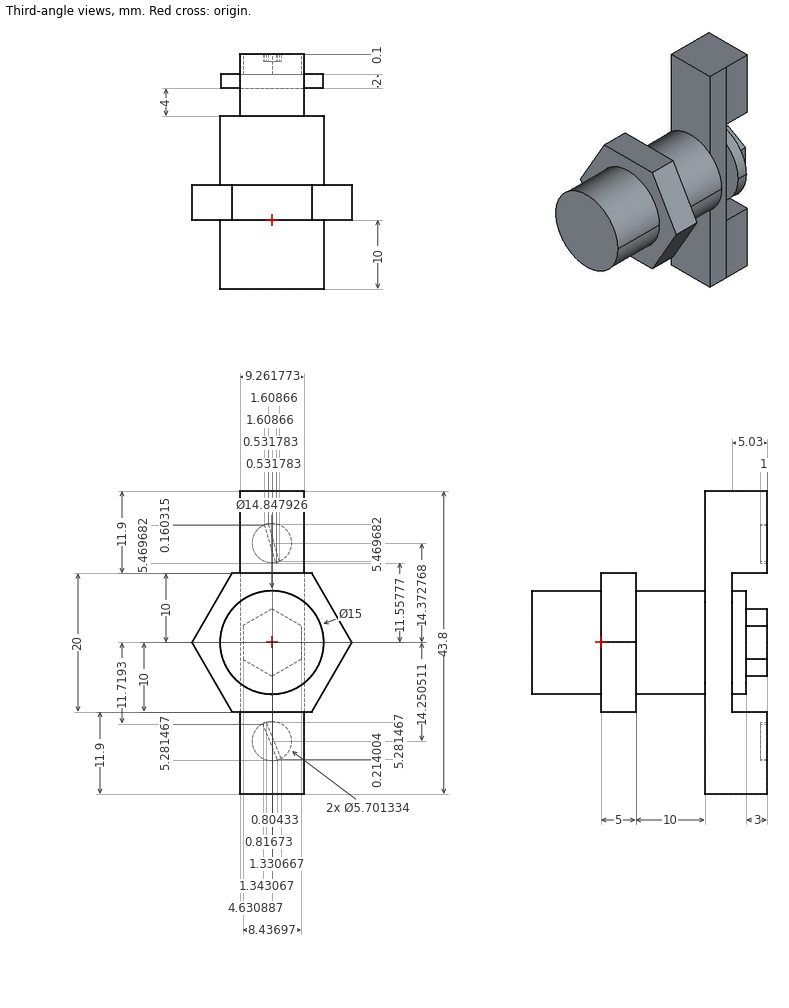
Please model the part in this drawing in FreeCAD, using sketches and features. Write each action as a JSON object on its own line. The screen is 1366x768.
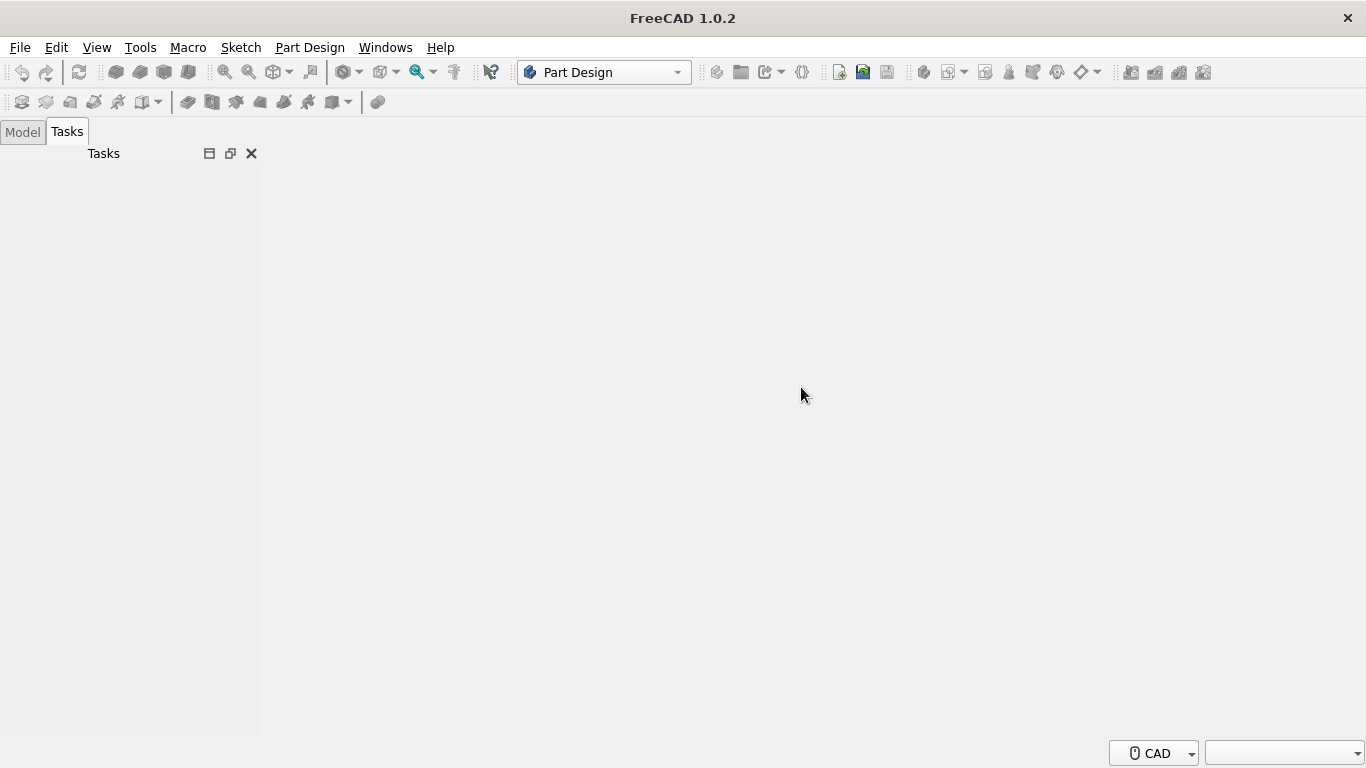
{"action": "left_click", "coordinate": [840, 72]}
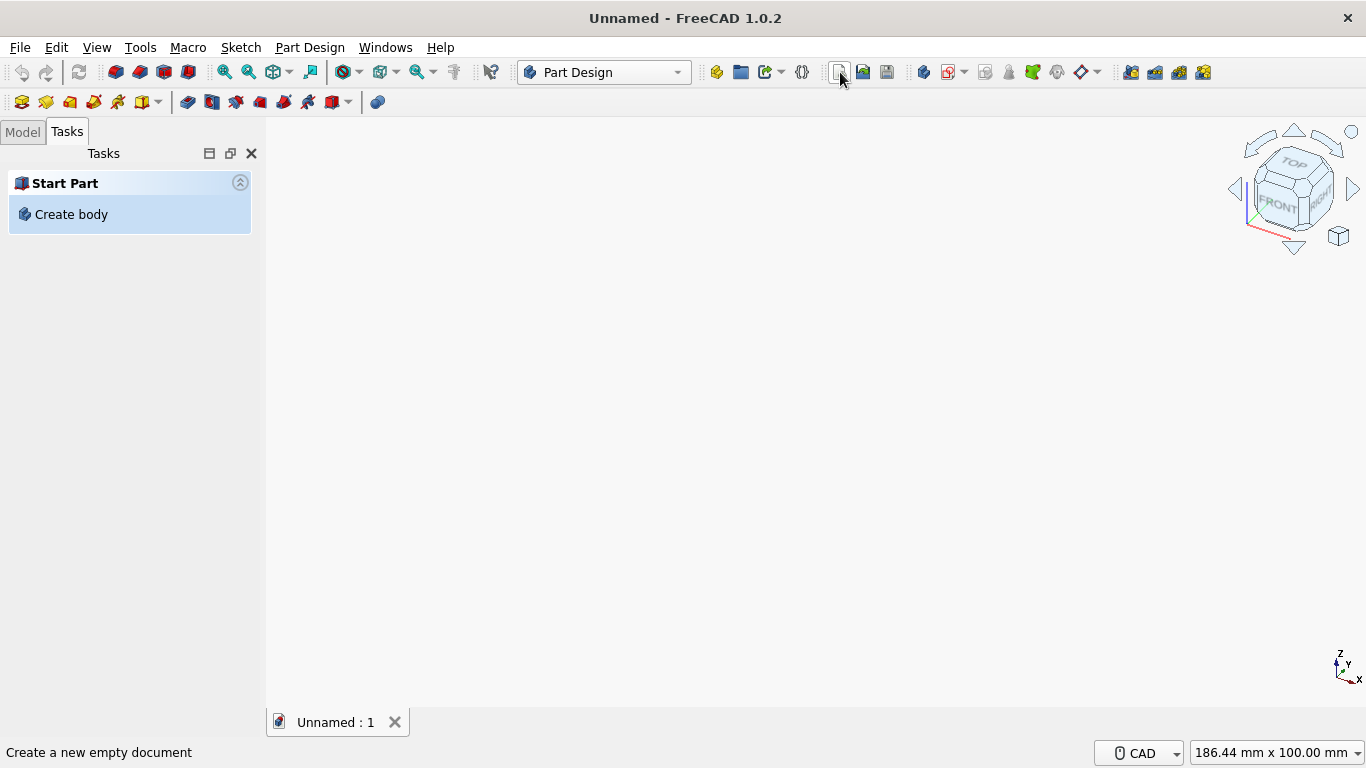
{"action": "left_click", "coordinate": [948, 72]}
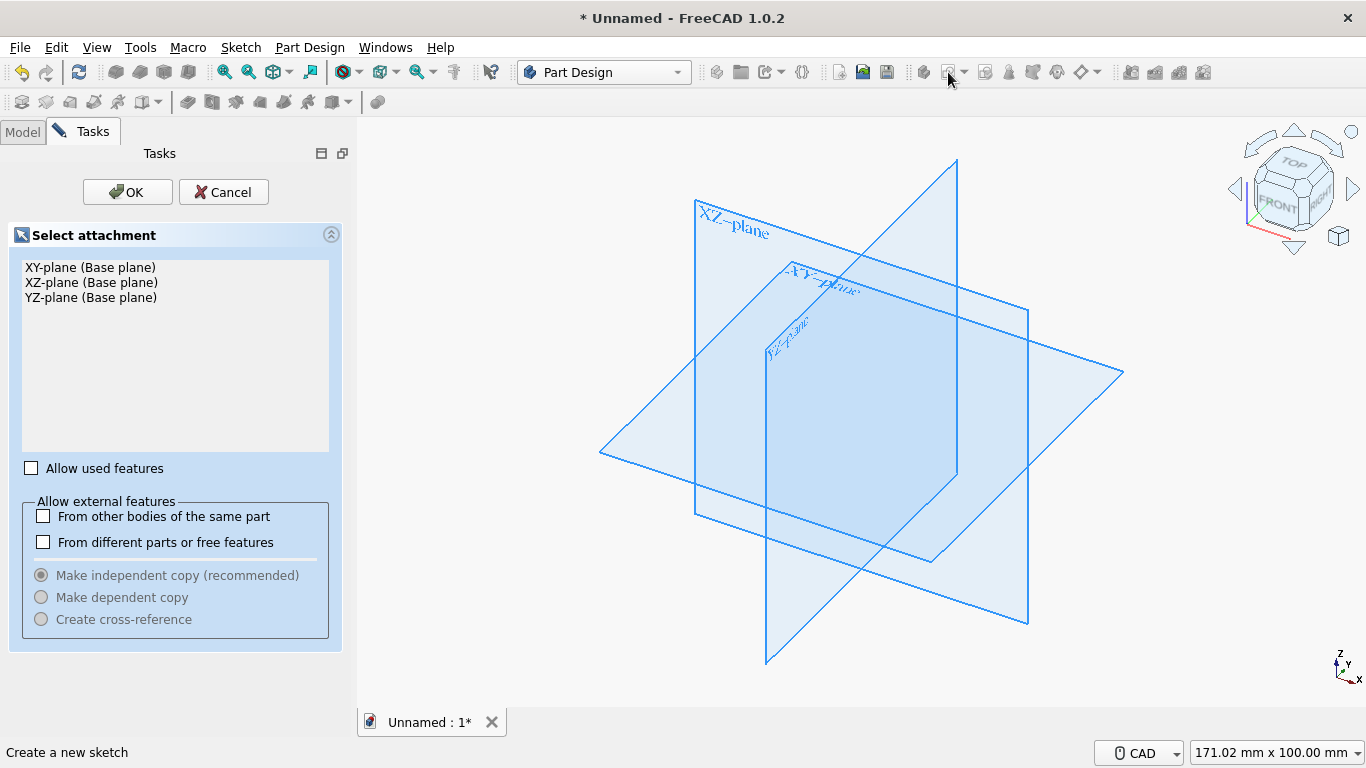
{"action": "left_click", "coordinate": [82, 282]}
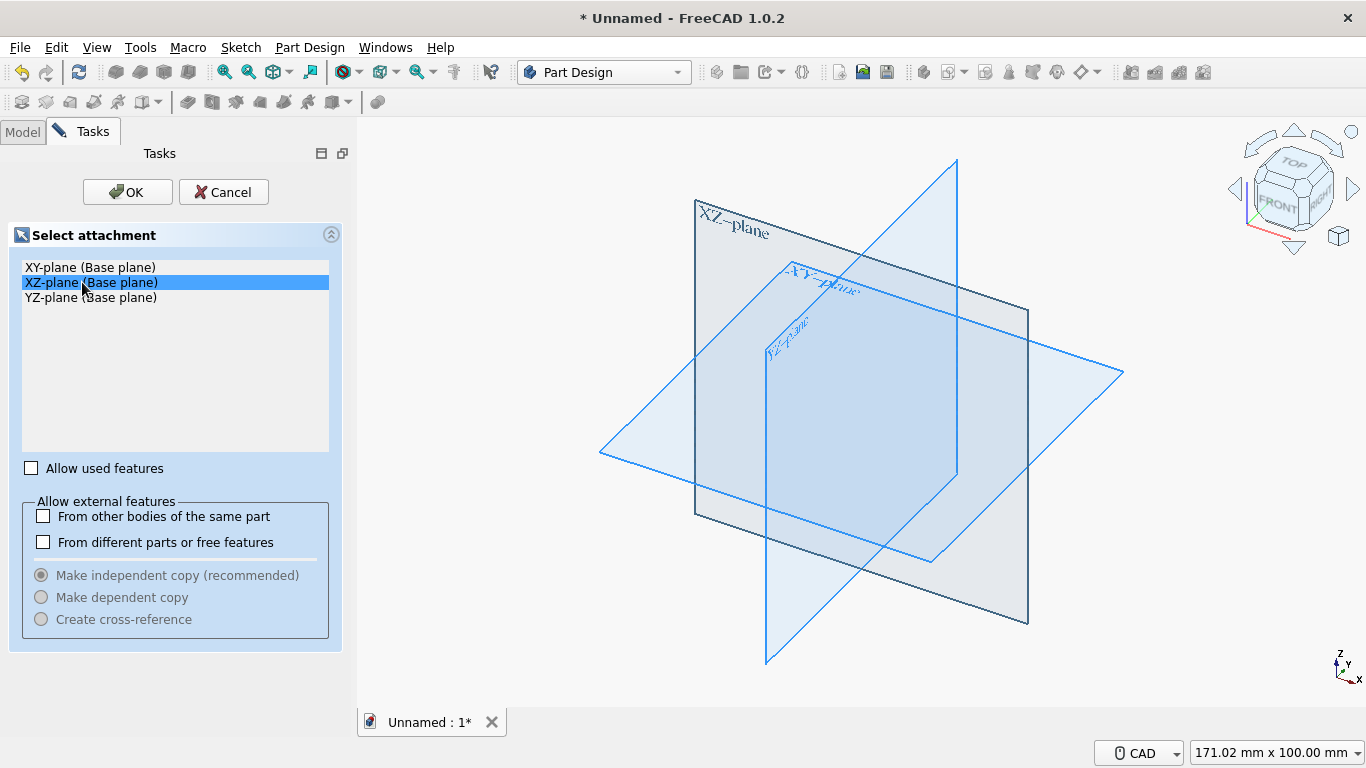
{"action": "left_click", "coordinate": [128, 192]}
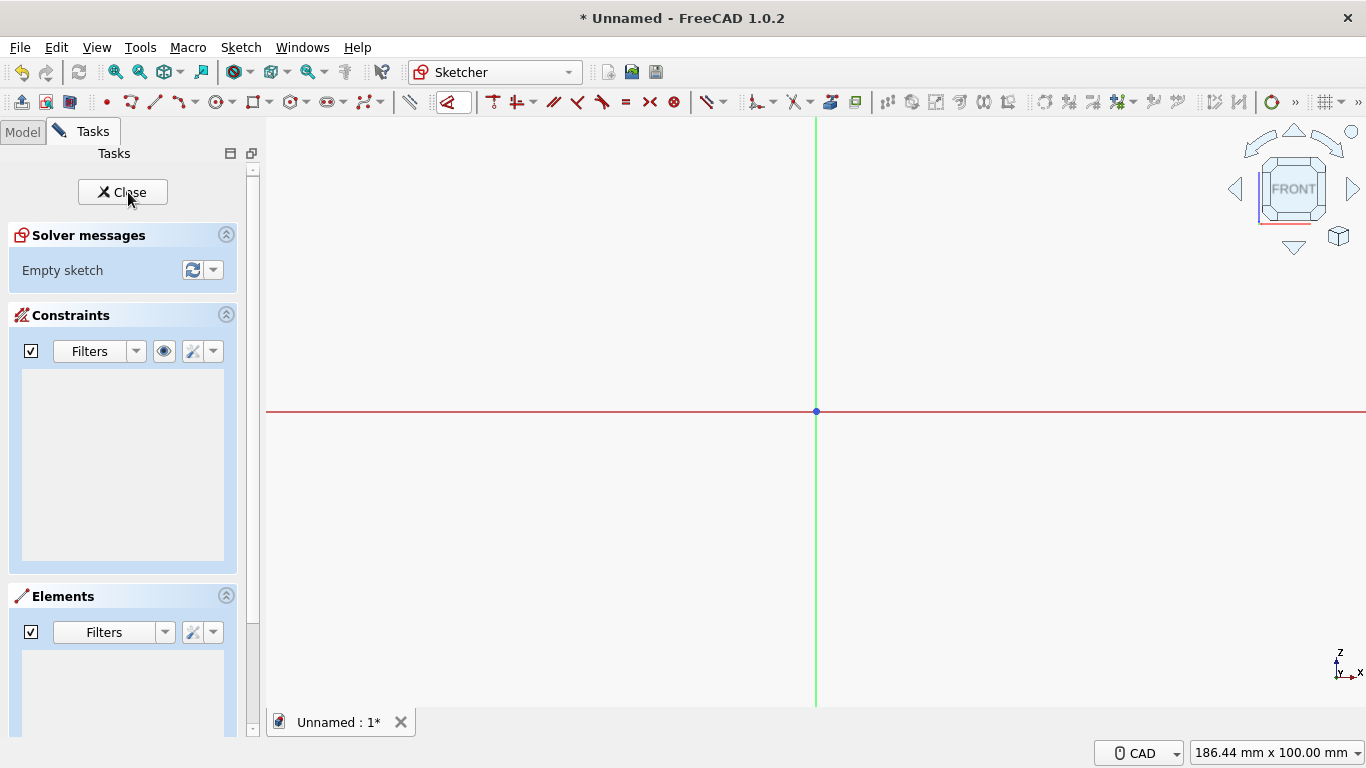
{"action": "scroll", "coordinate": [846, 412], "scroll_direction": "up", "scroll_amount": 6}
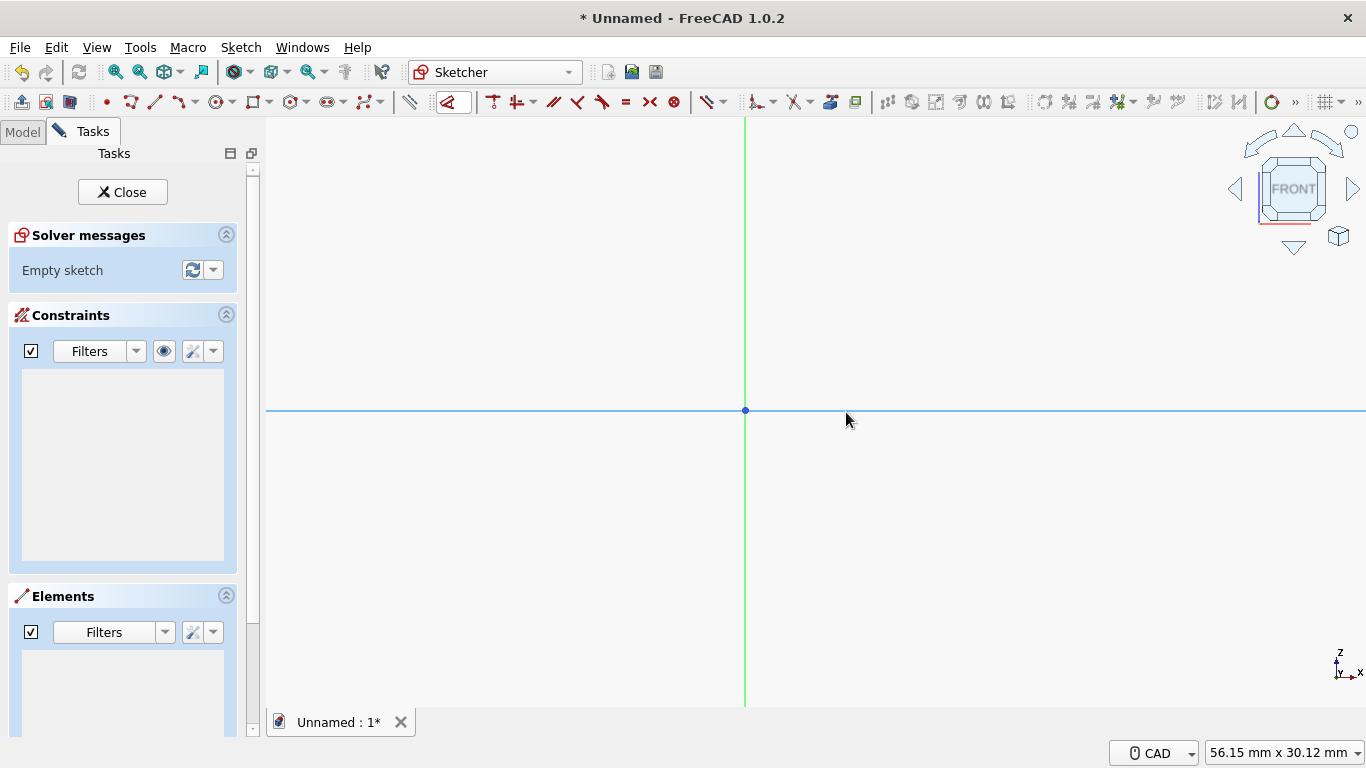
{"action": "left_click", "coordinate": [290, 102]}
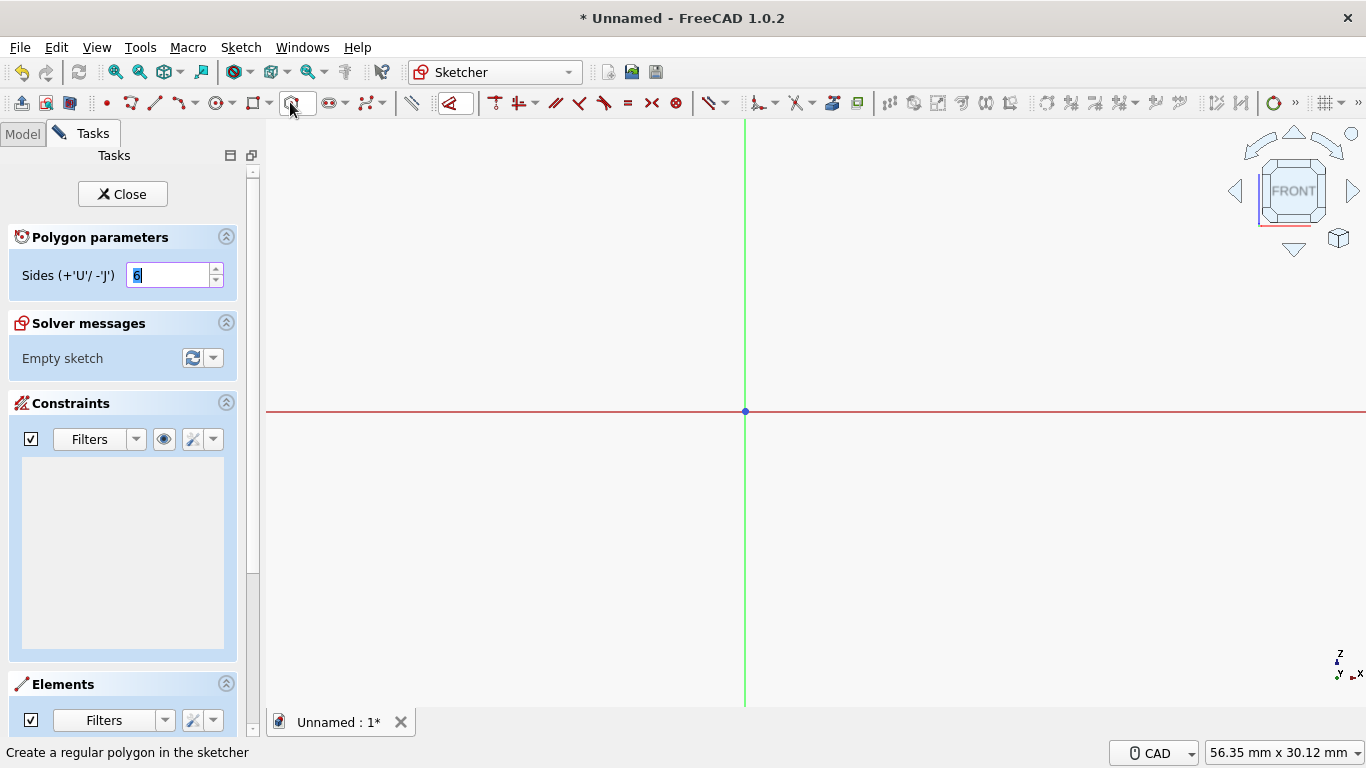
{"action": "left_click", "coordinate": [745, 412]}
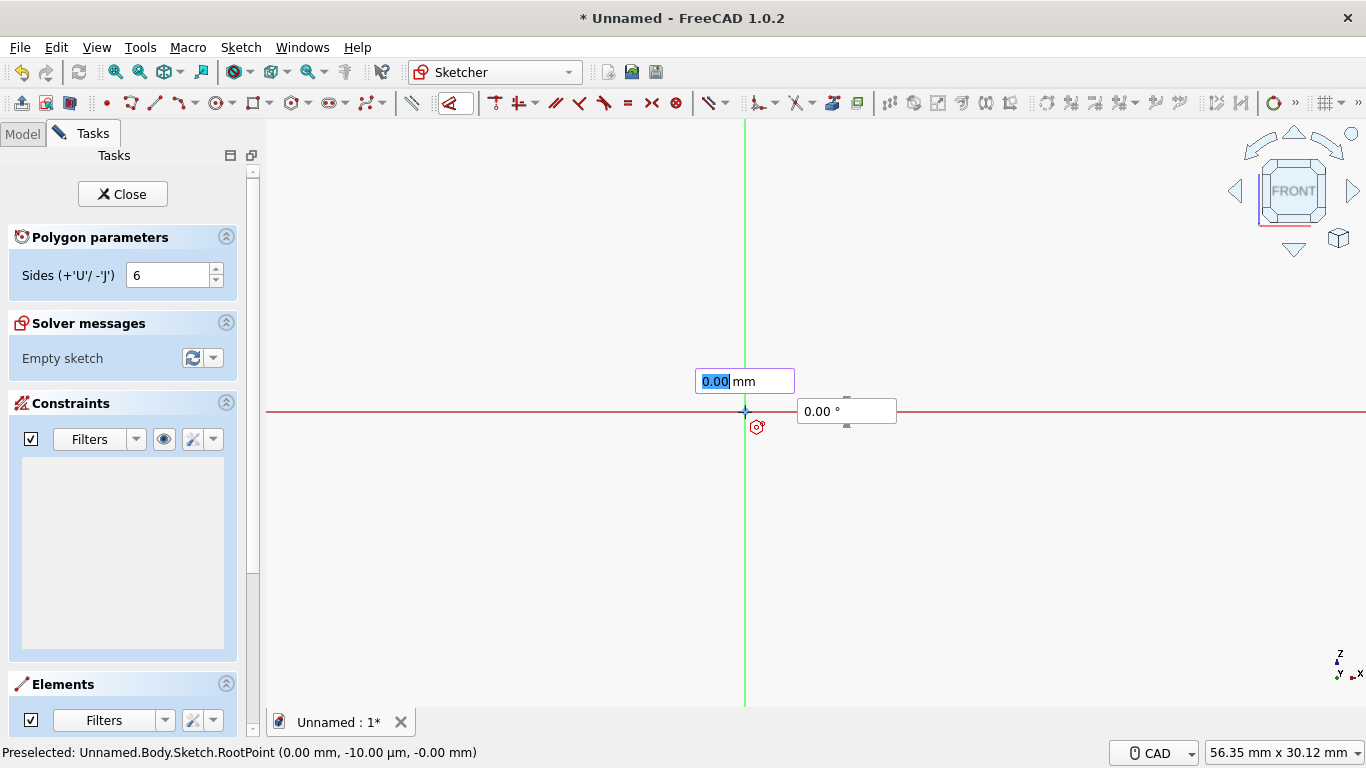
{"action": "left_click", "coordinate": [520, 412]}
{"action": "right_click", "coordinate": [520, 412]}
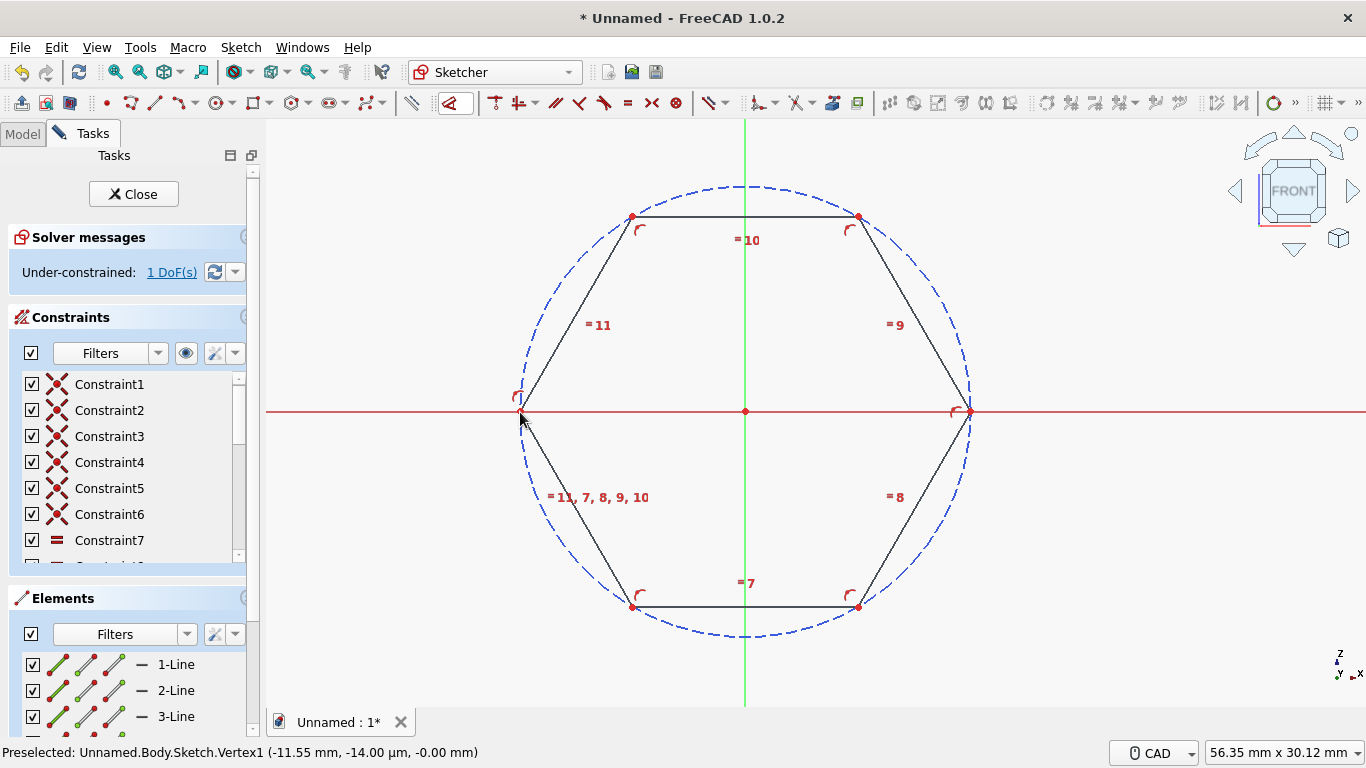
{"action": "left_click", "coordinate": [450, 104]}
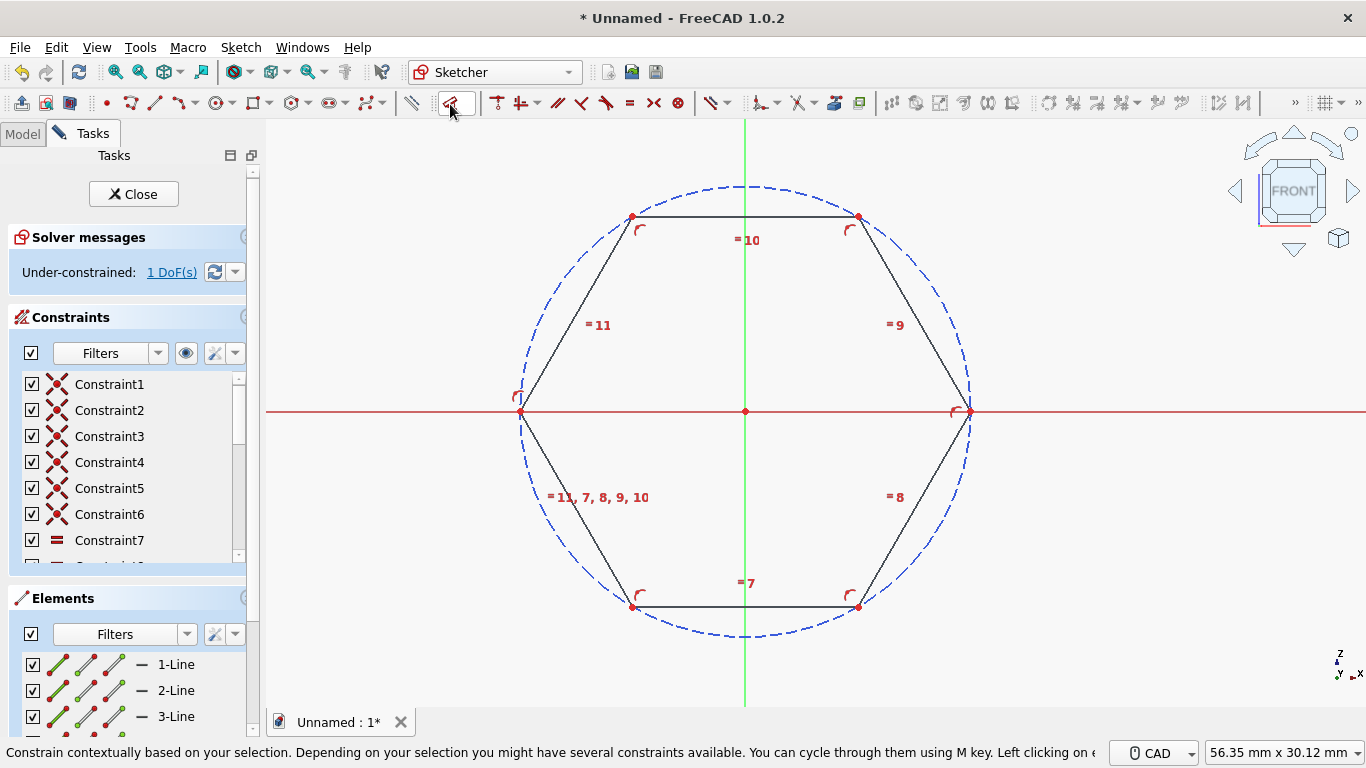
{"action": "left_click", "coordinate": [633, 607]}